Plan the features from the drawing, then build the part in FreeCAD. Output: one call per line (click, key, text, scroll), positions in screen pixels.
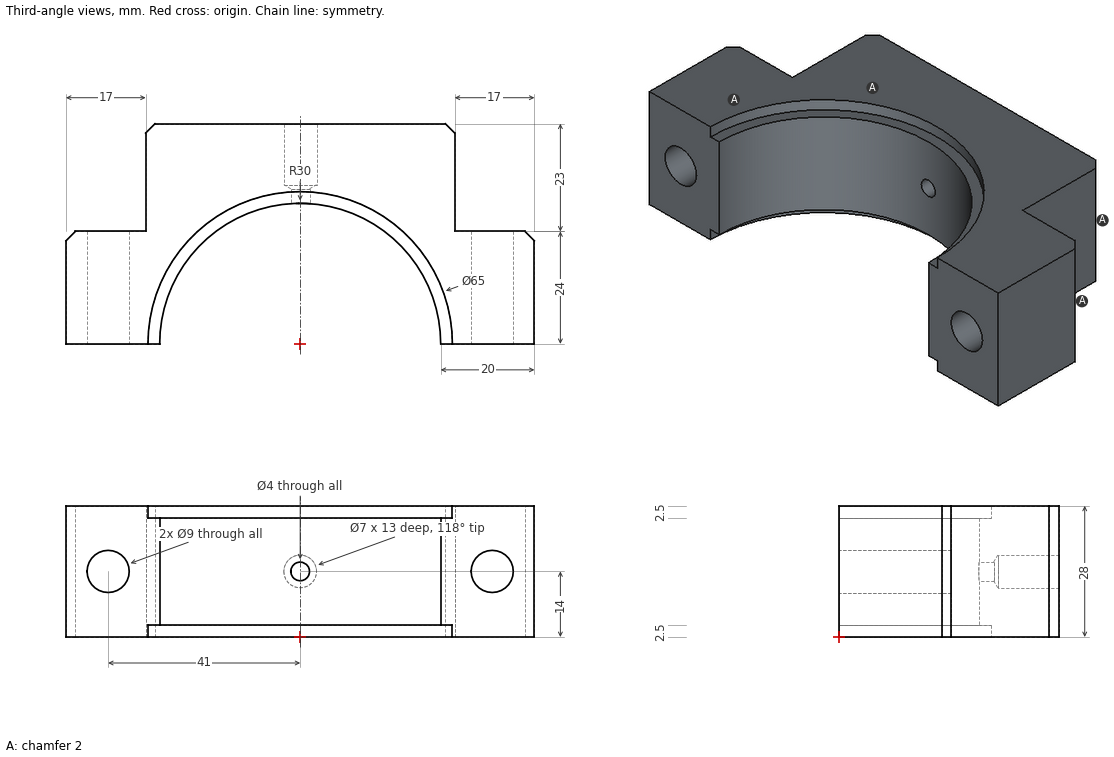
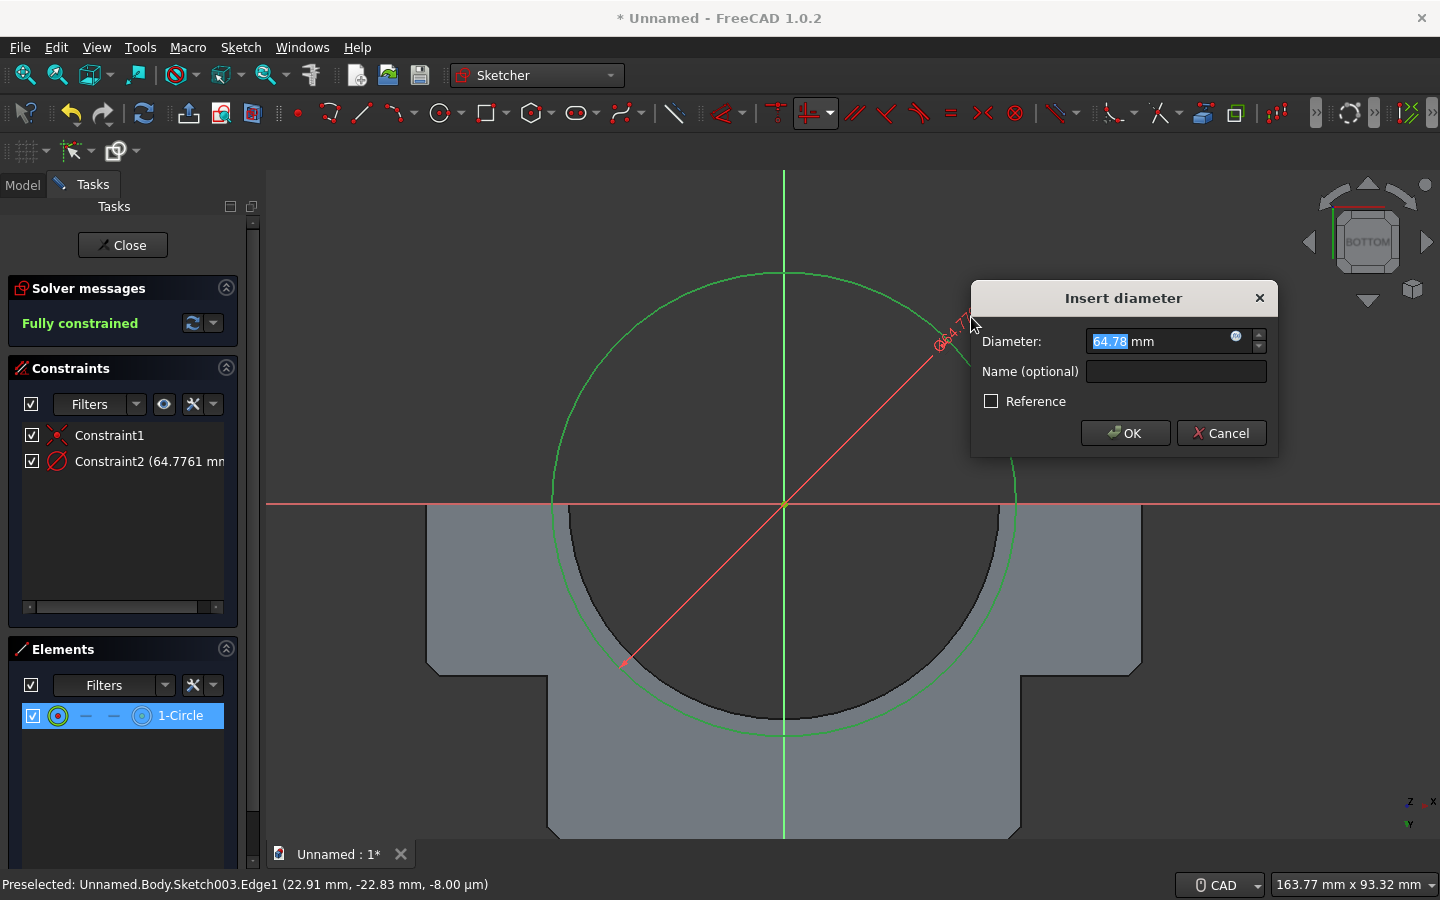
text(65)
key(Return)
key(Escape)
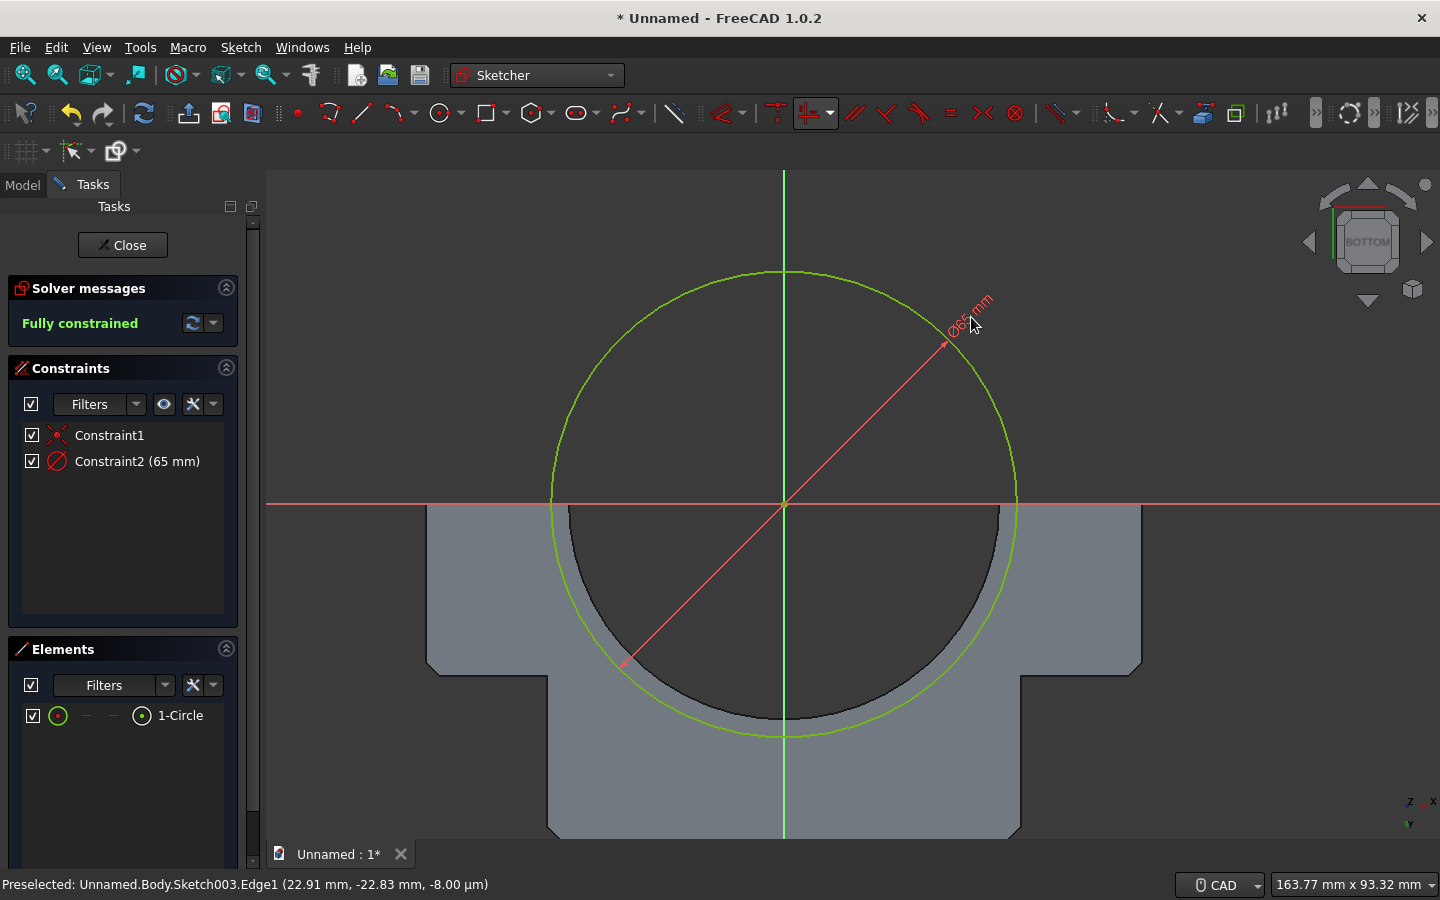
click(123, 245)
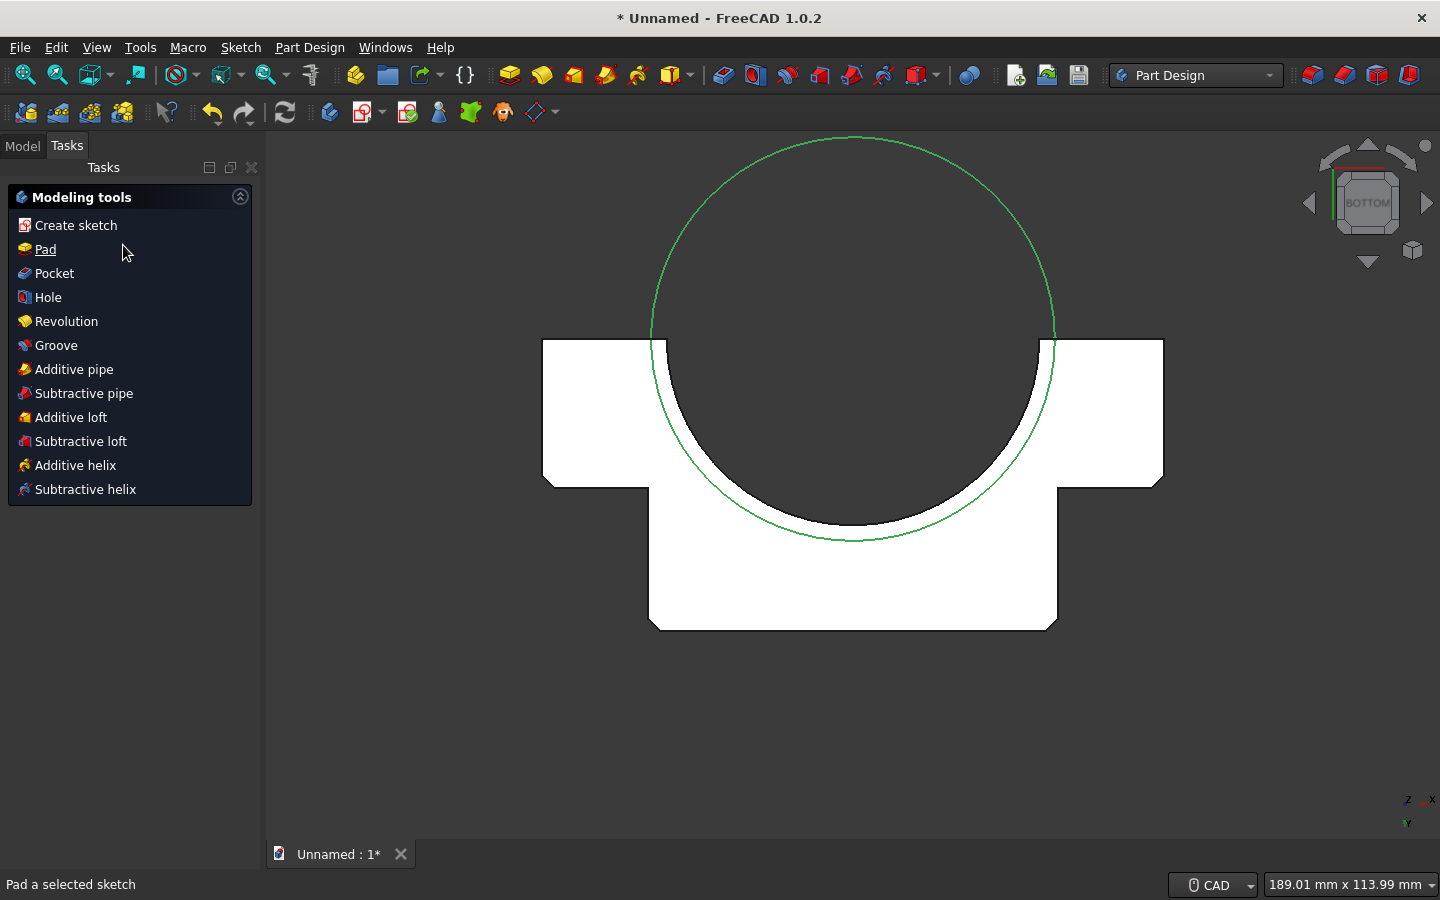
click(724, 76)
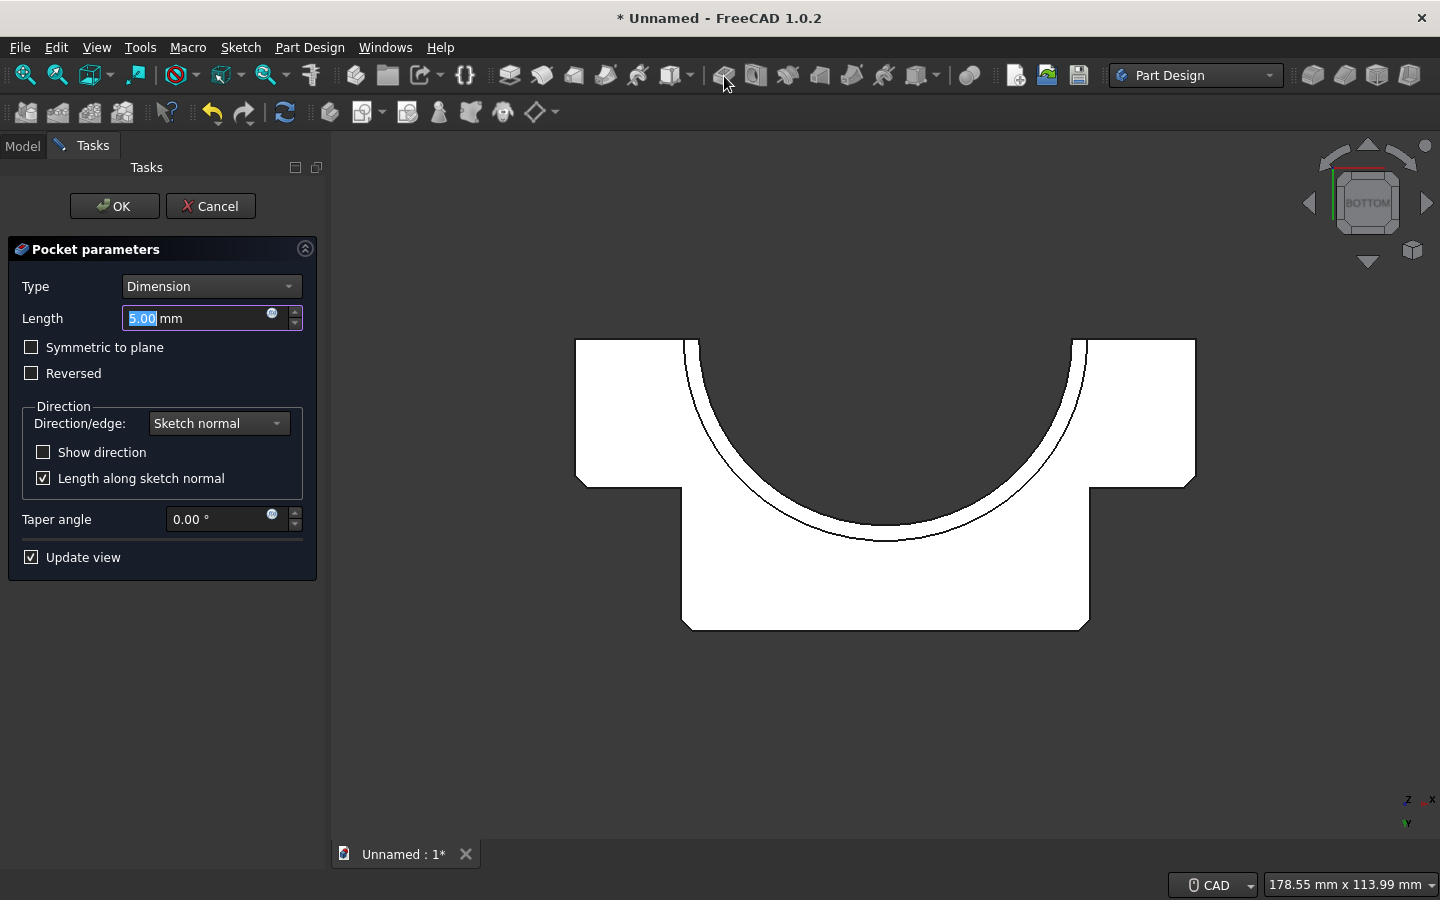
text(2.5)
key(Tab)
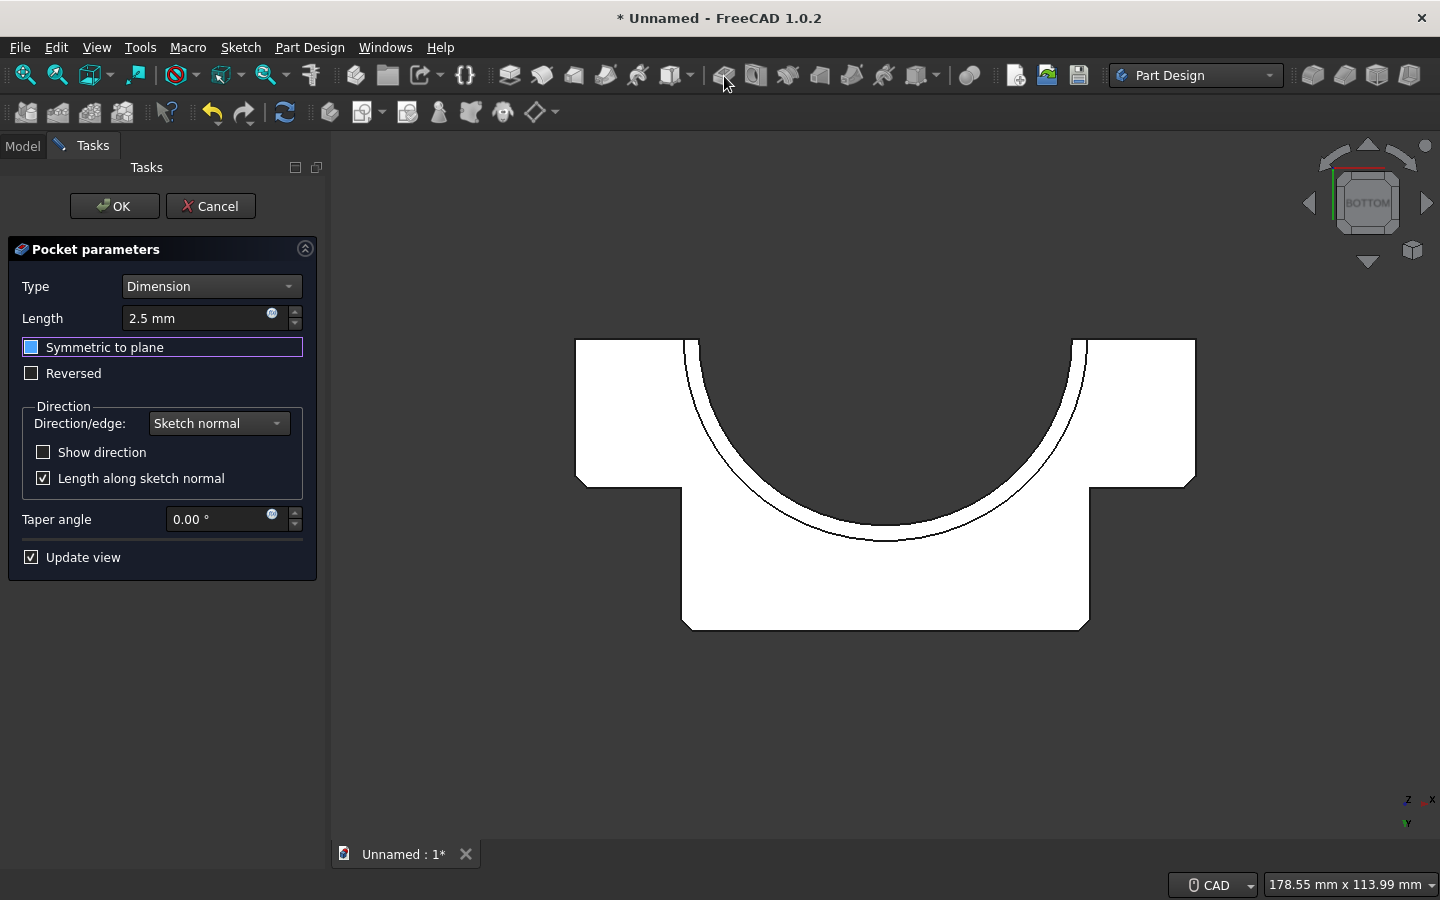
click(115, 206)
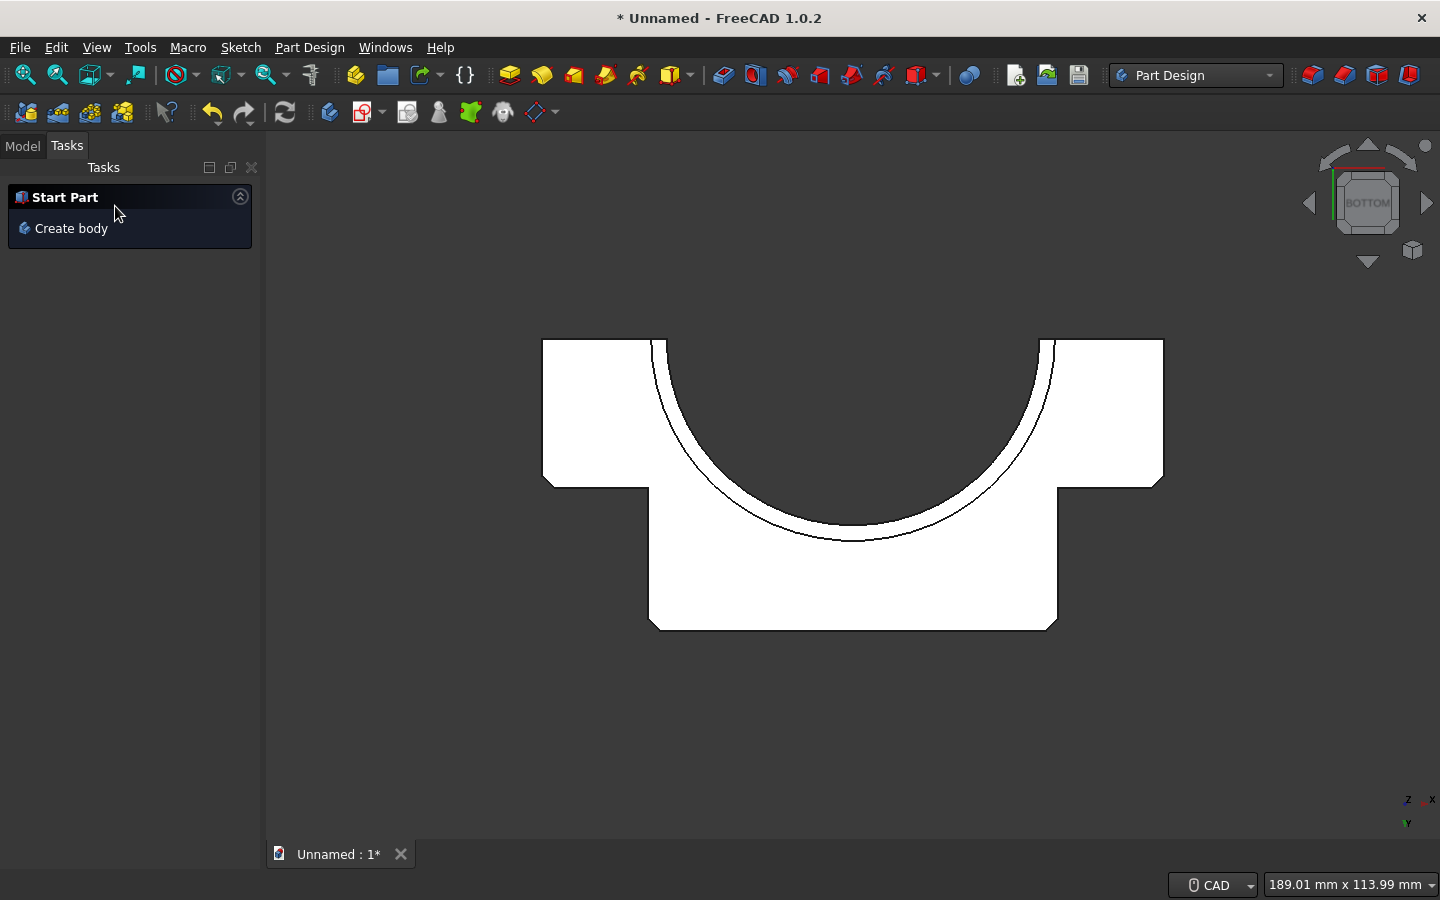
click(23, 145)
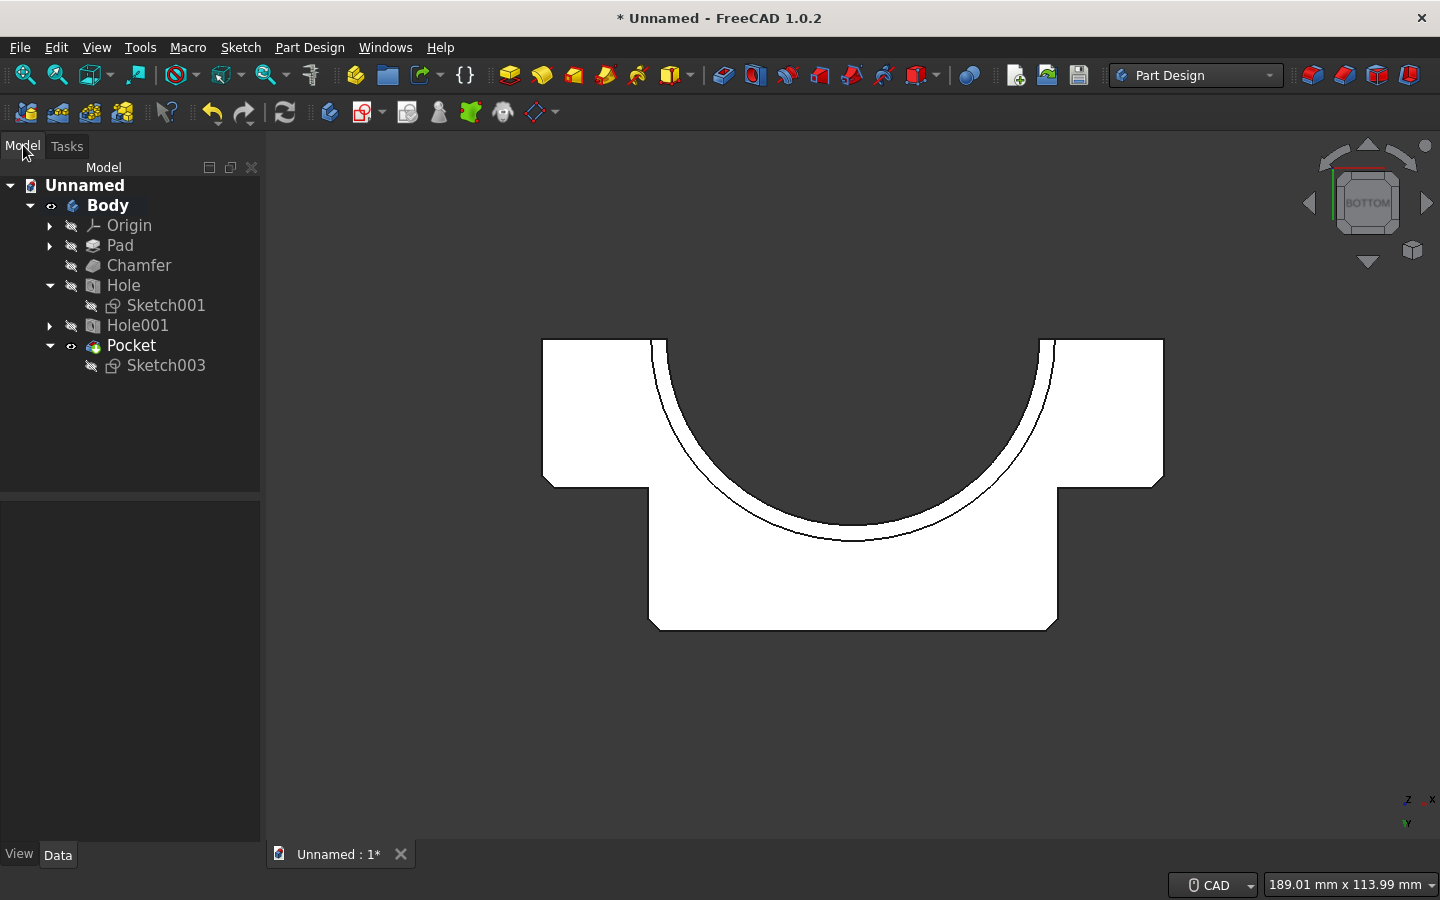
click(50, 226)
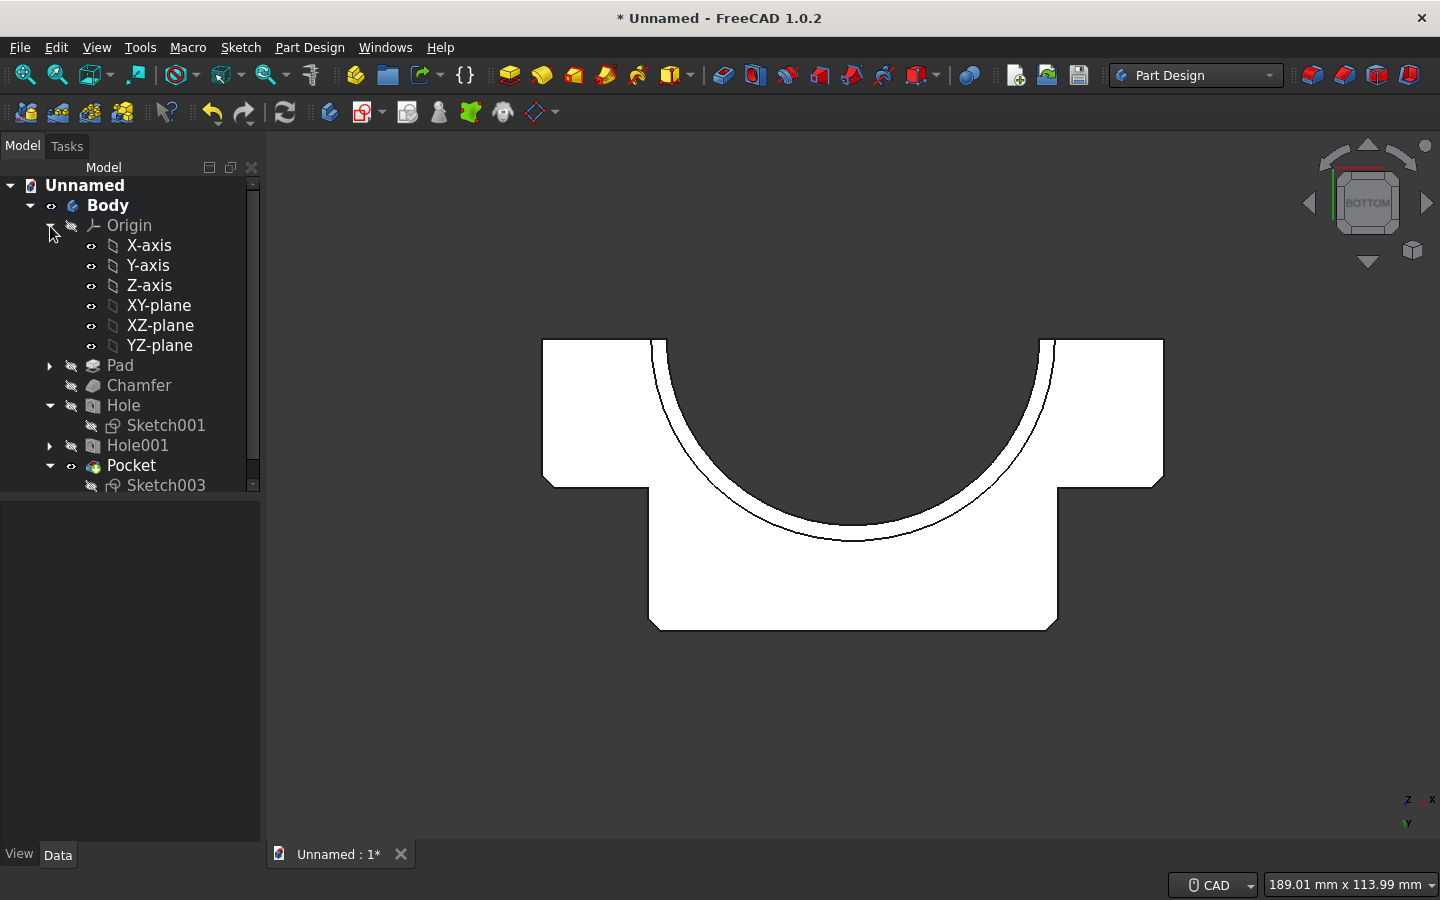
click(136, 306)